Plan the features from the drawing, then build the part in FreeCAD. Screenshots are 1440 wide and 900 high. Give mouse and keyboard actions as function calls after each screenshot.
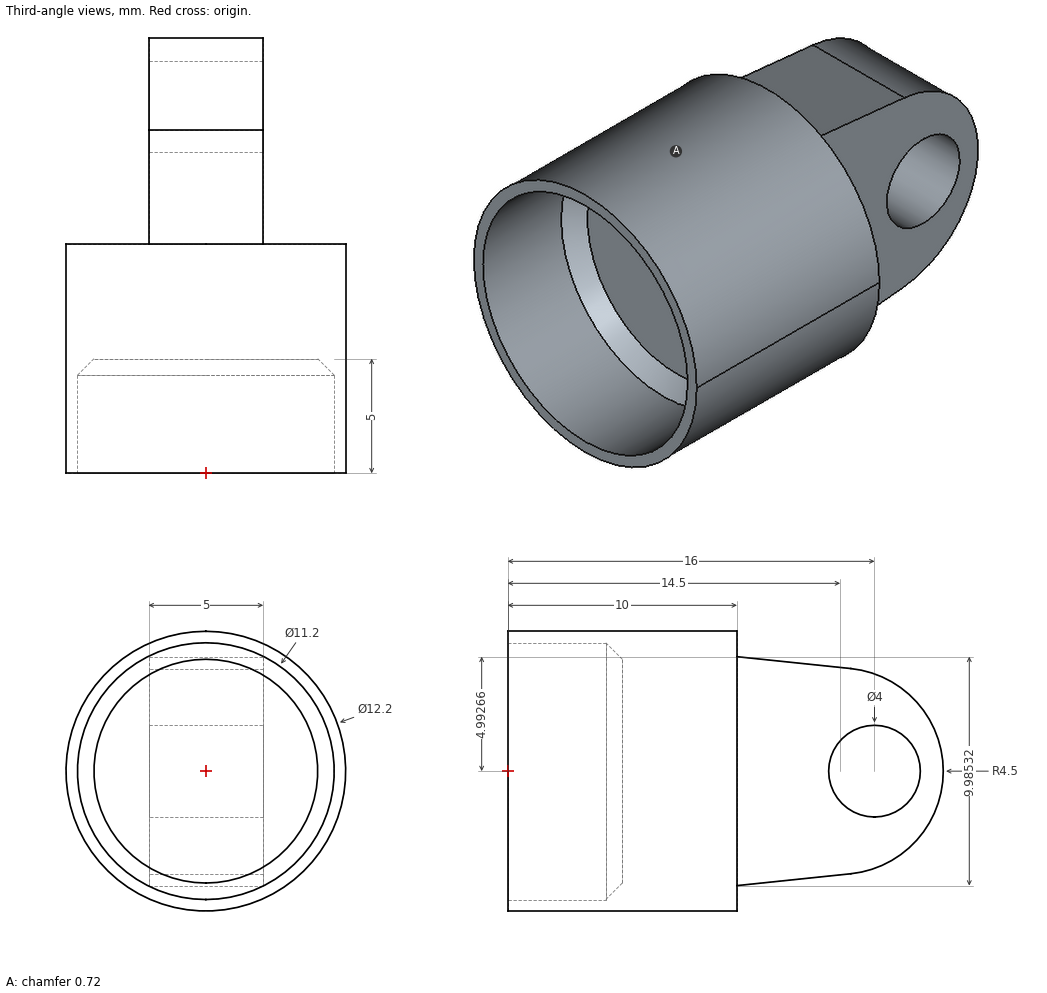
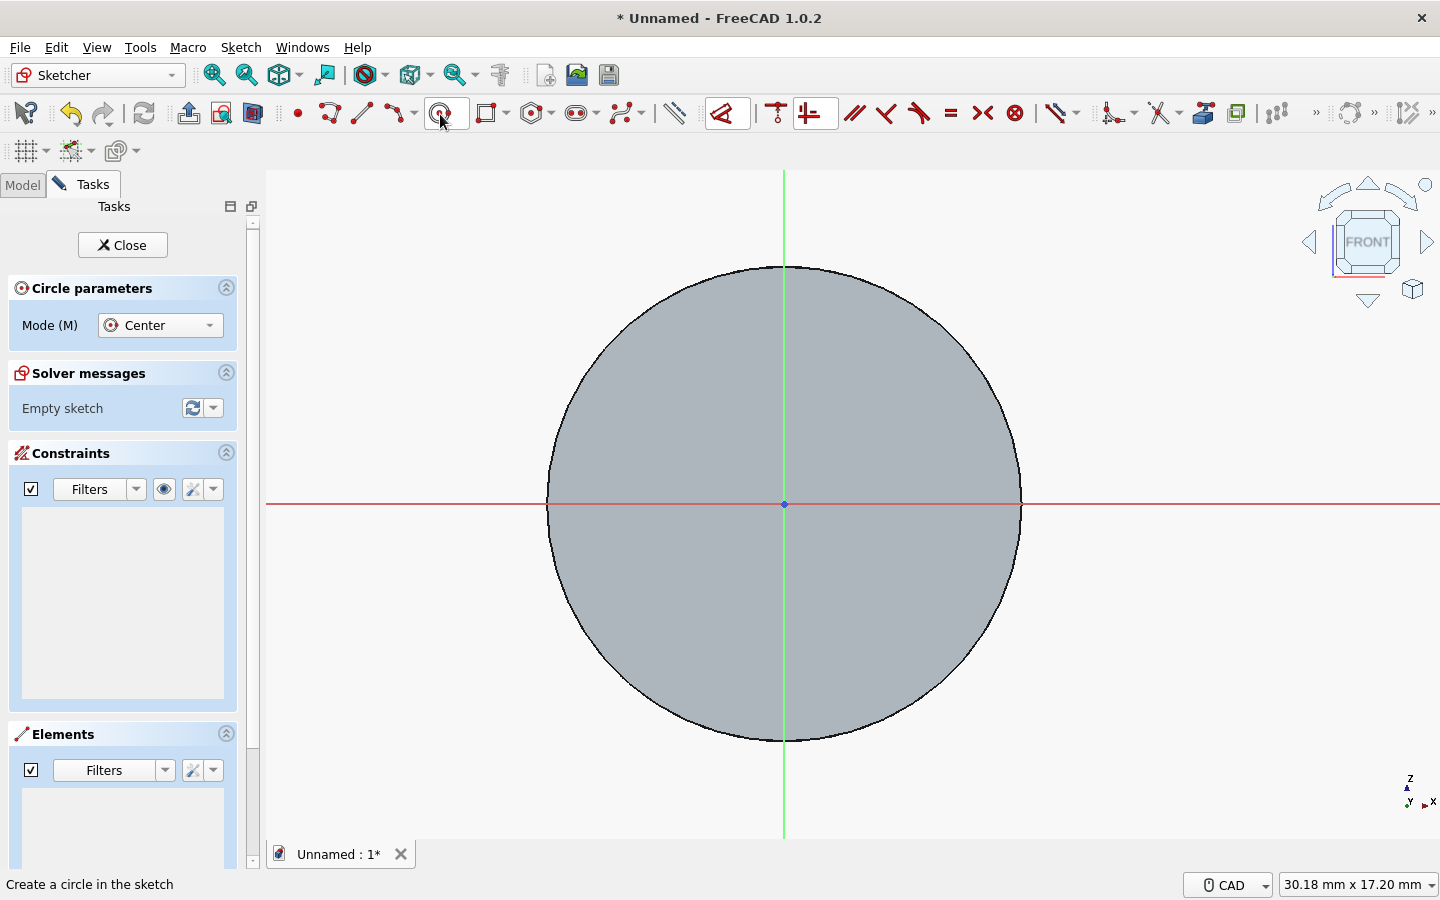
click(784, 504)
click(938, 350)
key(Escape)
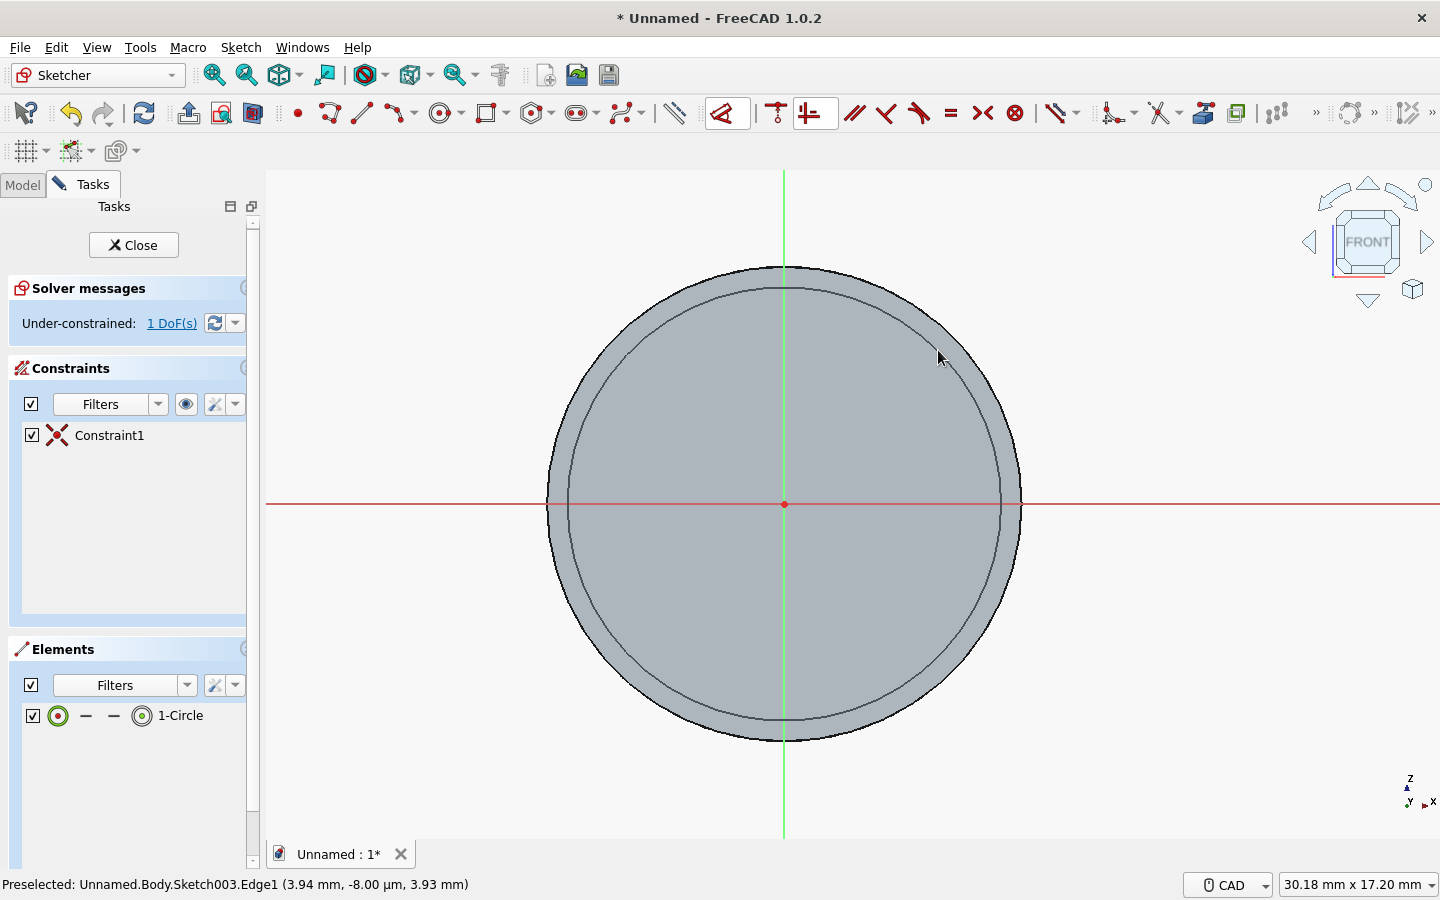
key(d)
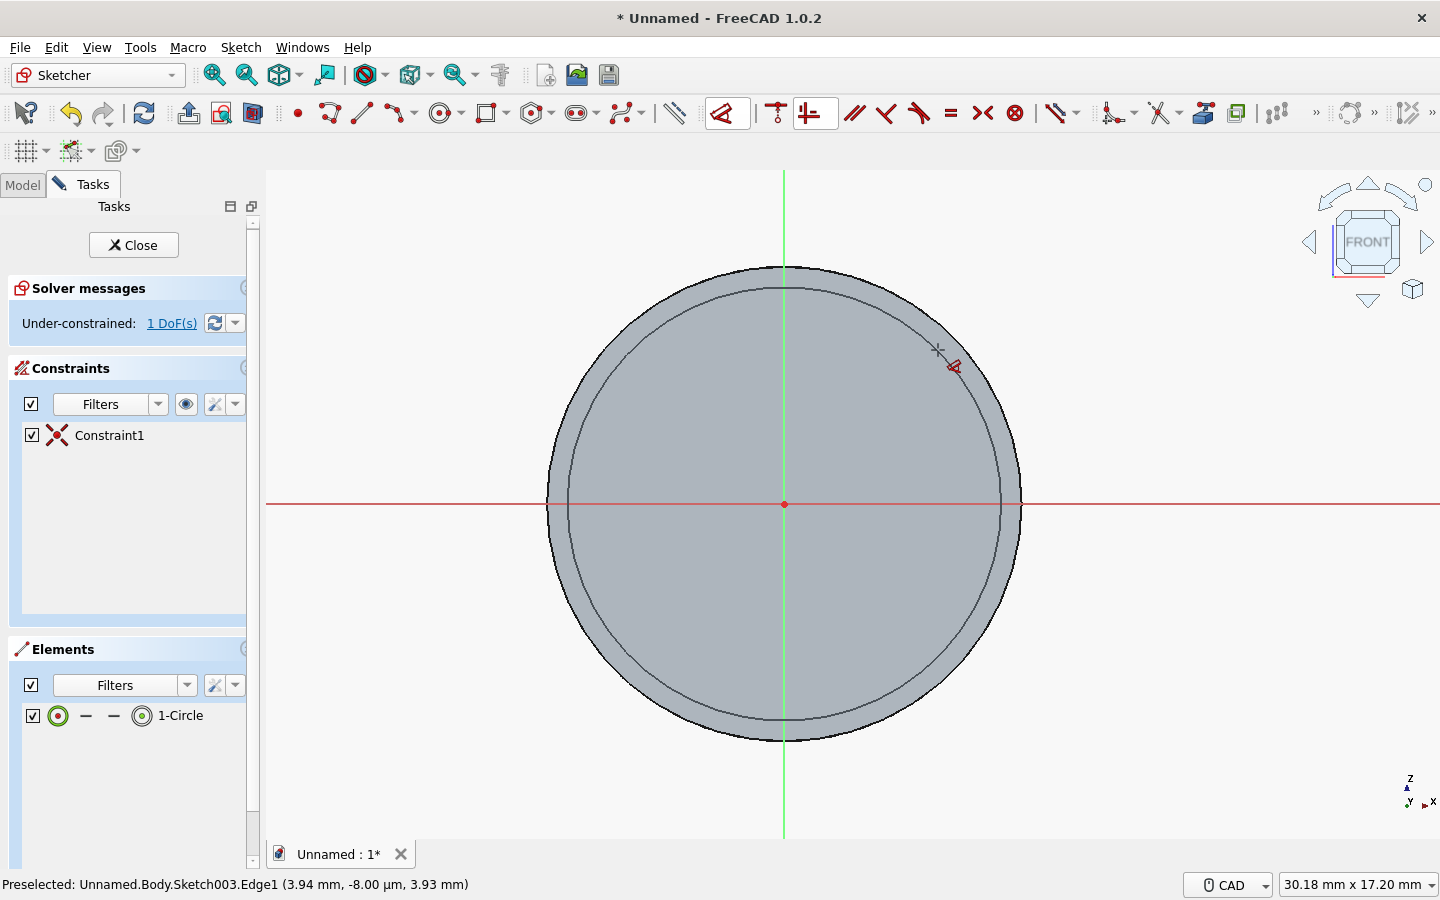
click(937, 350)
click(960, 327)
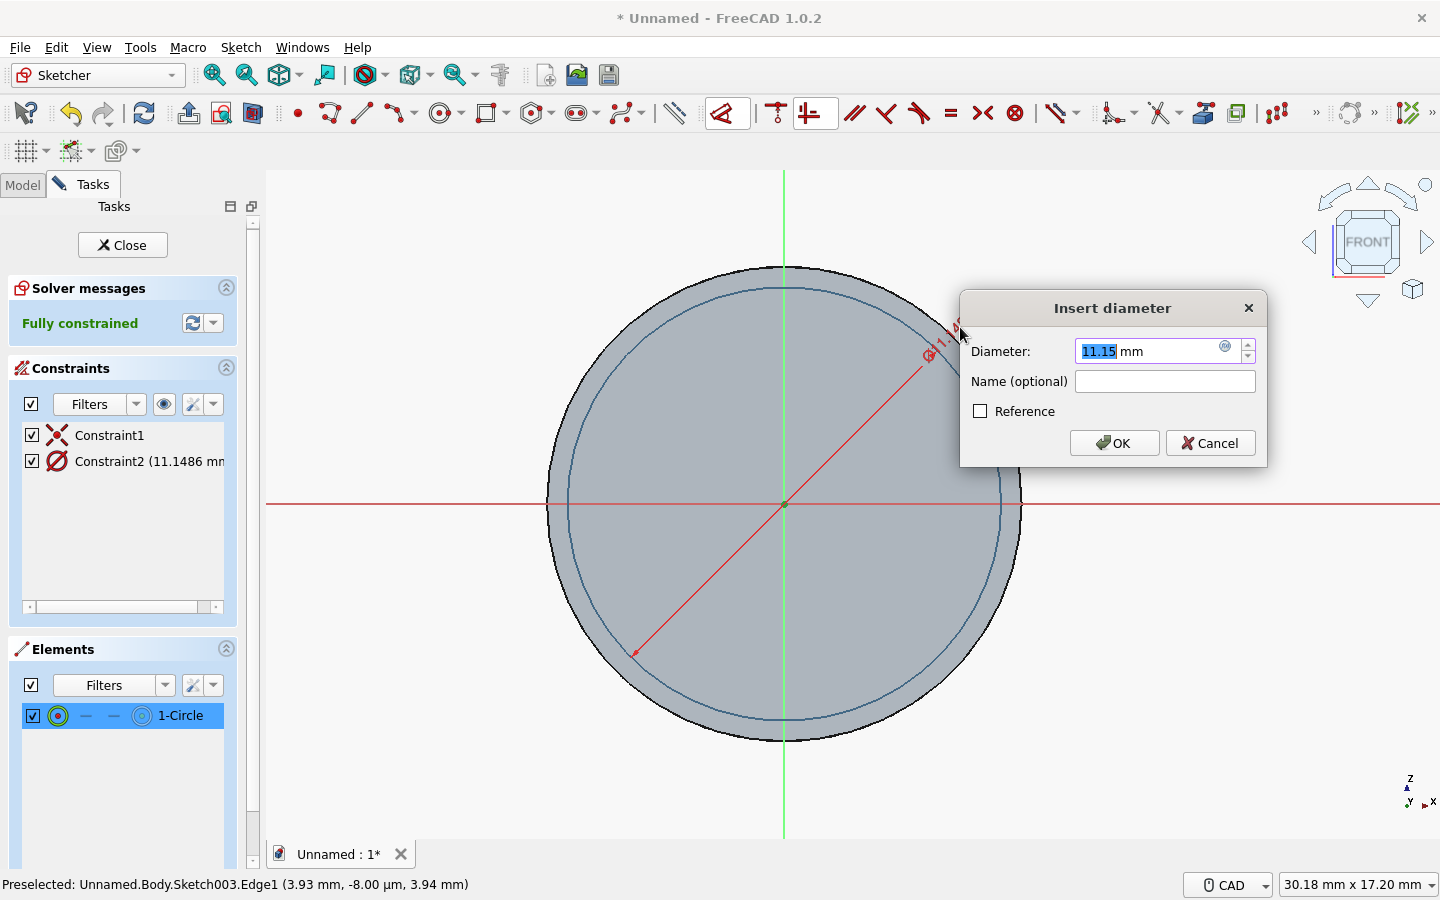
text(11.2)
key(Return)
key(Escape)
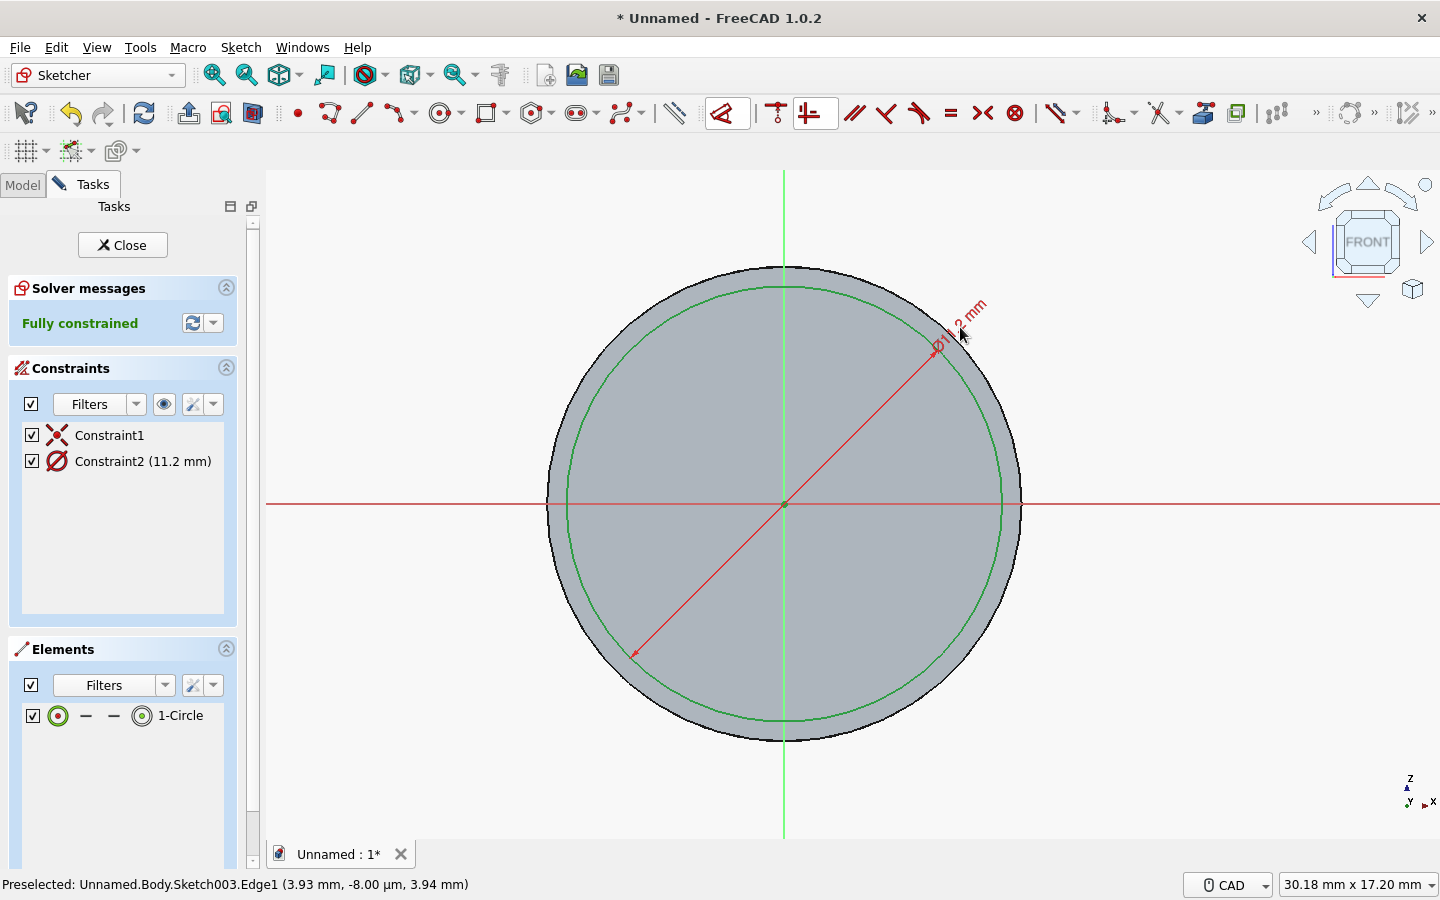
click(123, 245)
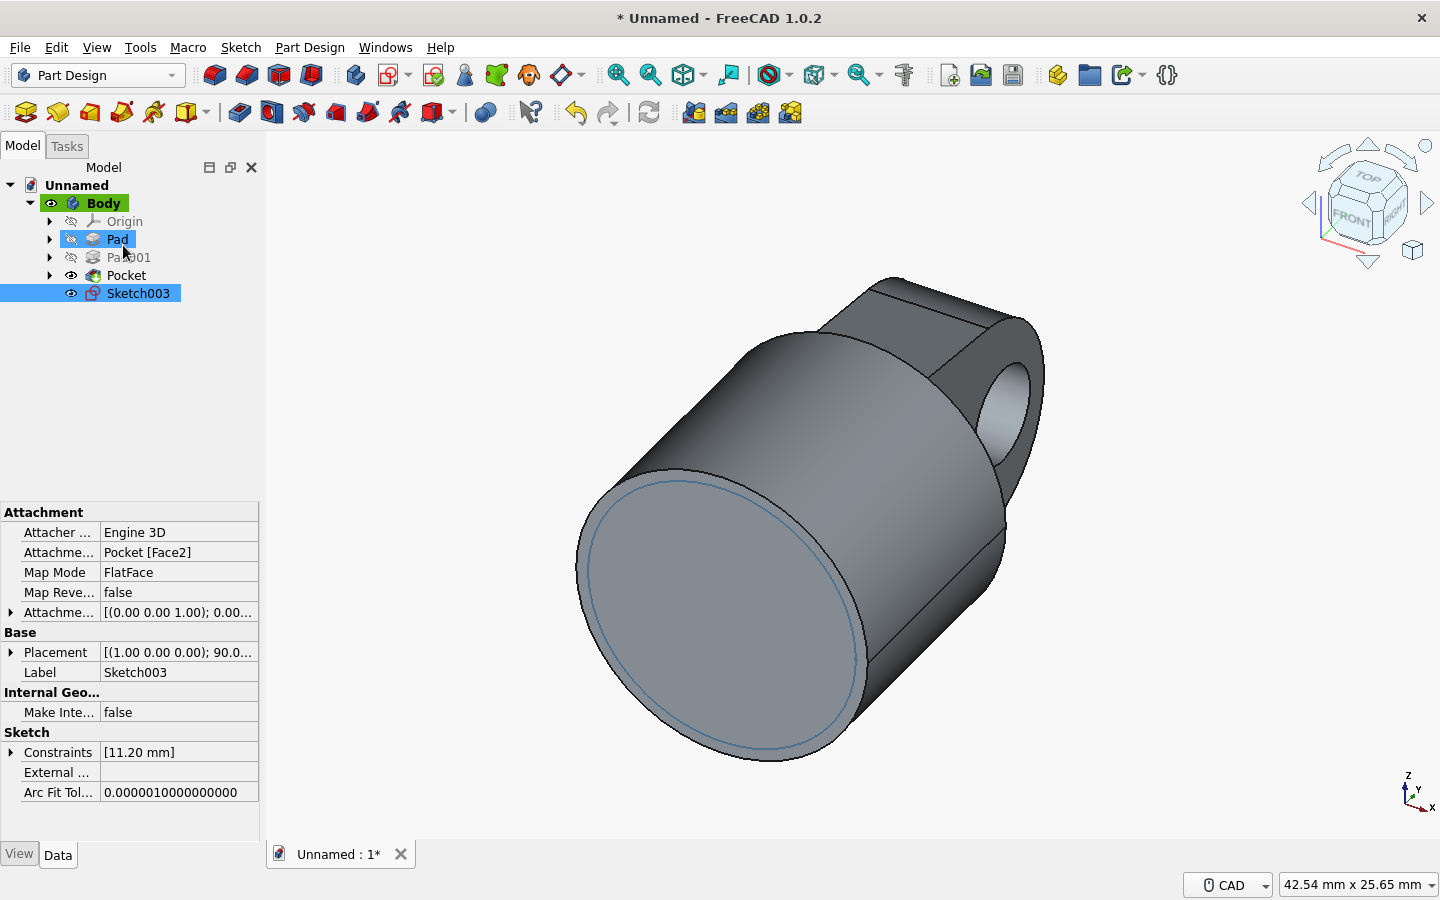
click(240, 112)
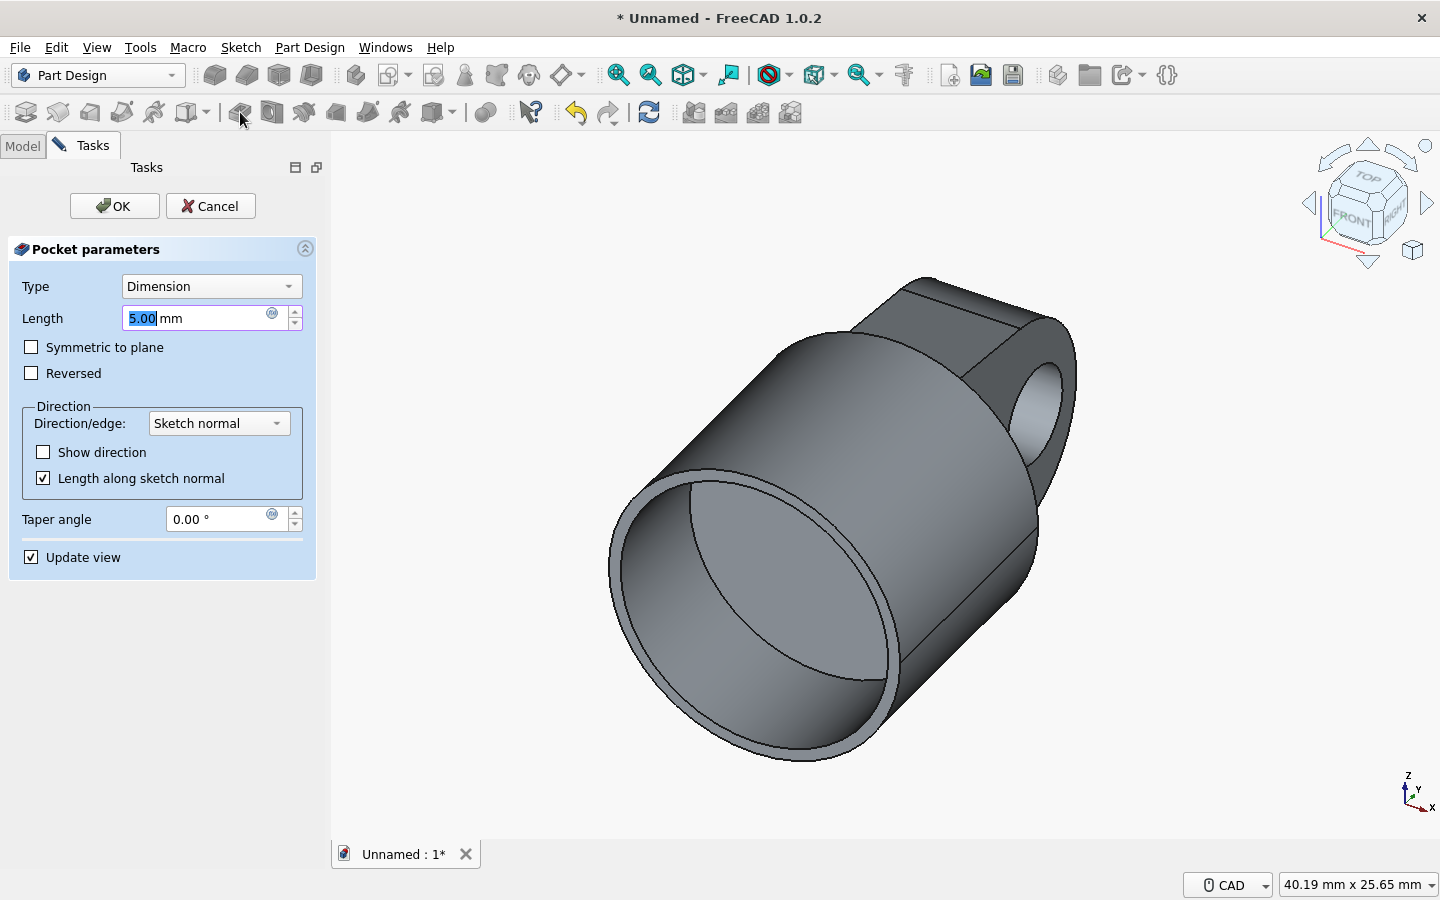
text(5)
key(Tab)